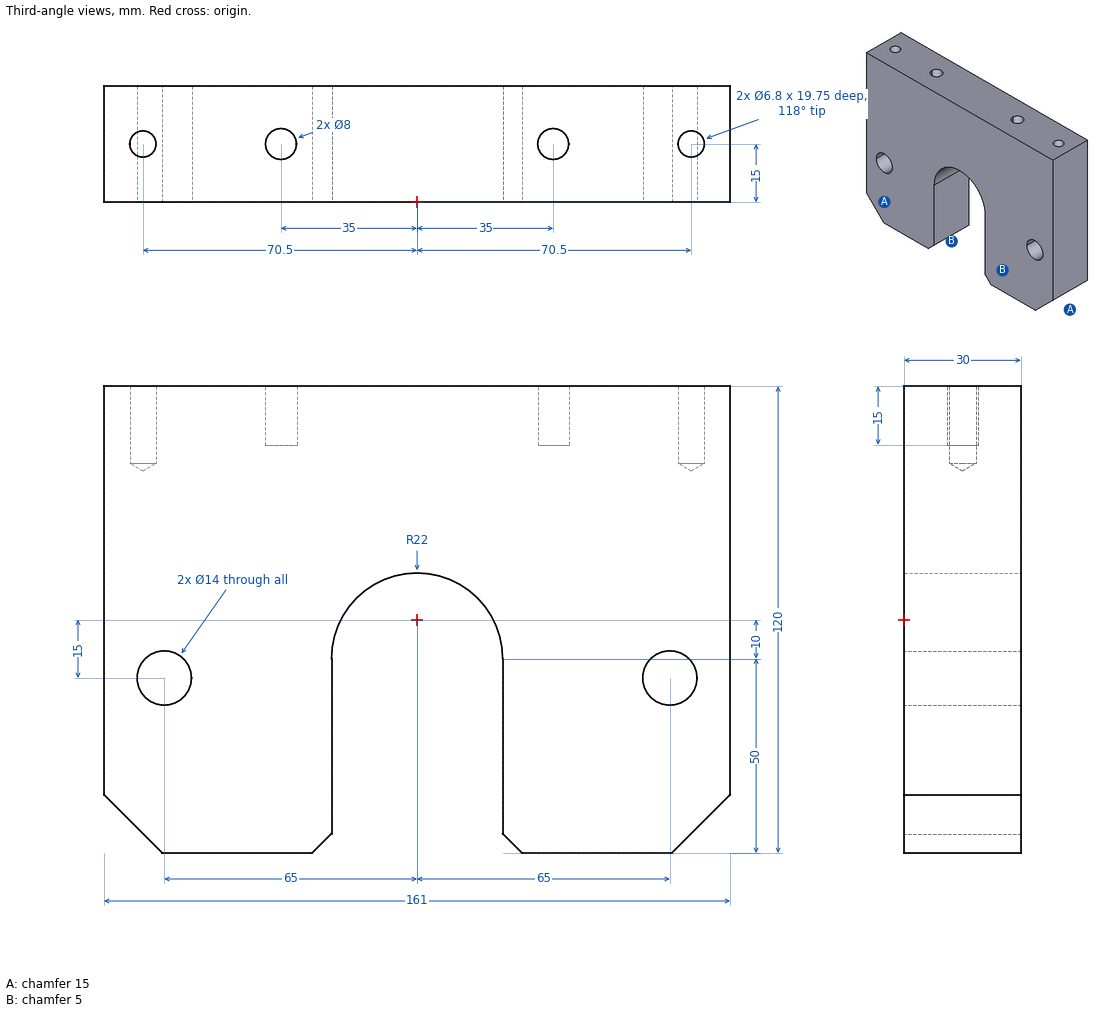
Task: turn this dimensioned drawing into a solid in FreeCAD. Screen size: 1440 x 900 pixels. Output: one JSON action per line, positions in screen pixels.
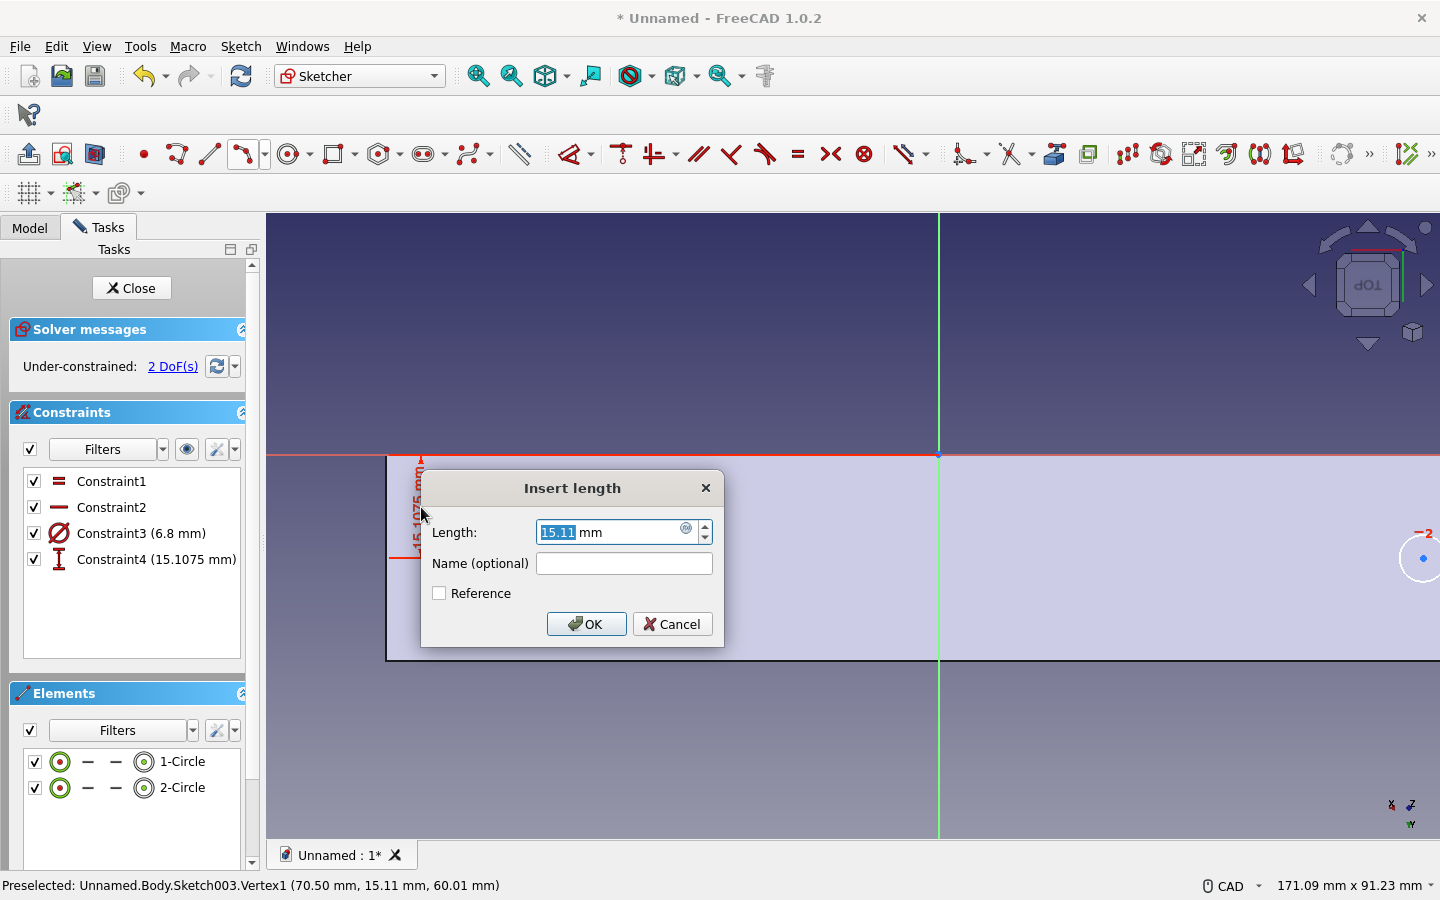
{"action": "type", "text": "15"}
{"action": "key", "text": "Return"}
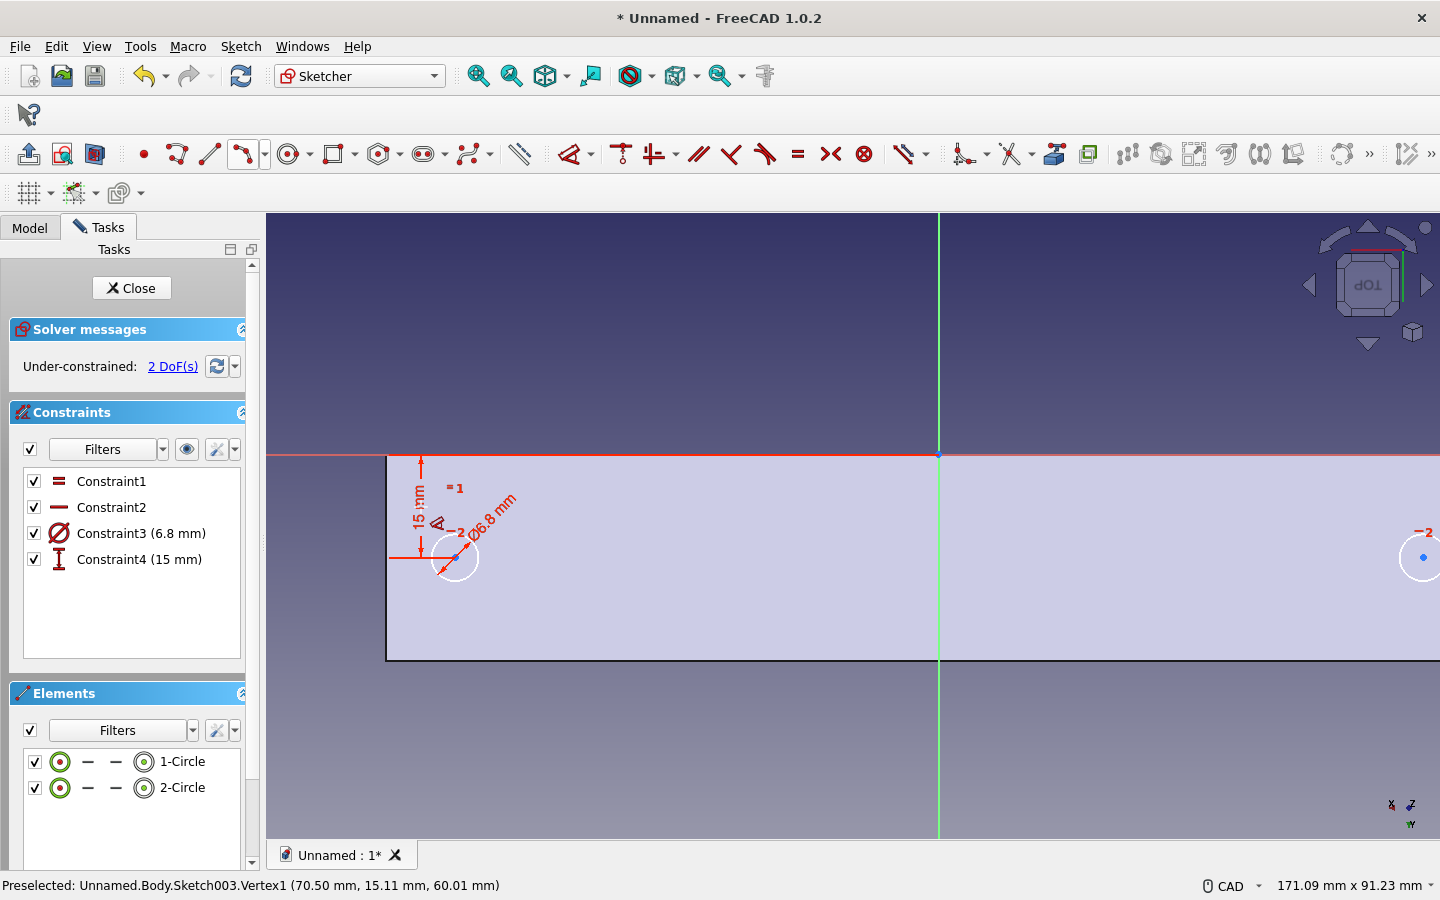
{"action": "left_click", "coordinate": [455, 558]}
{"action": "left_click", "coordinate": [697, 421]}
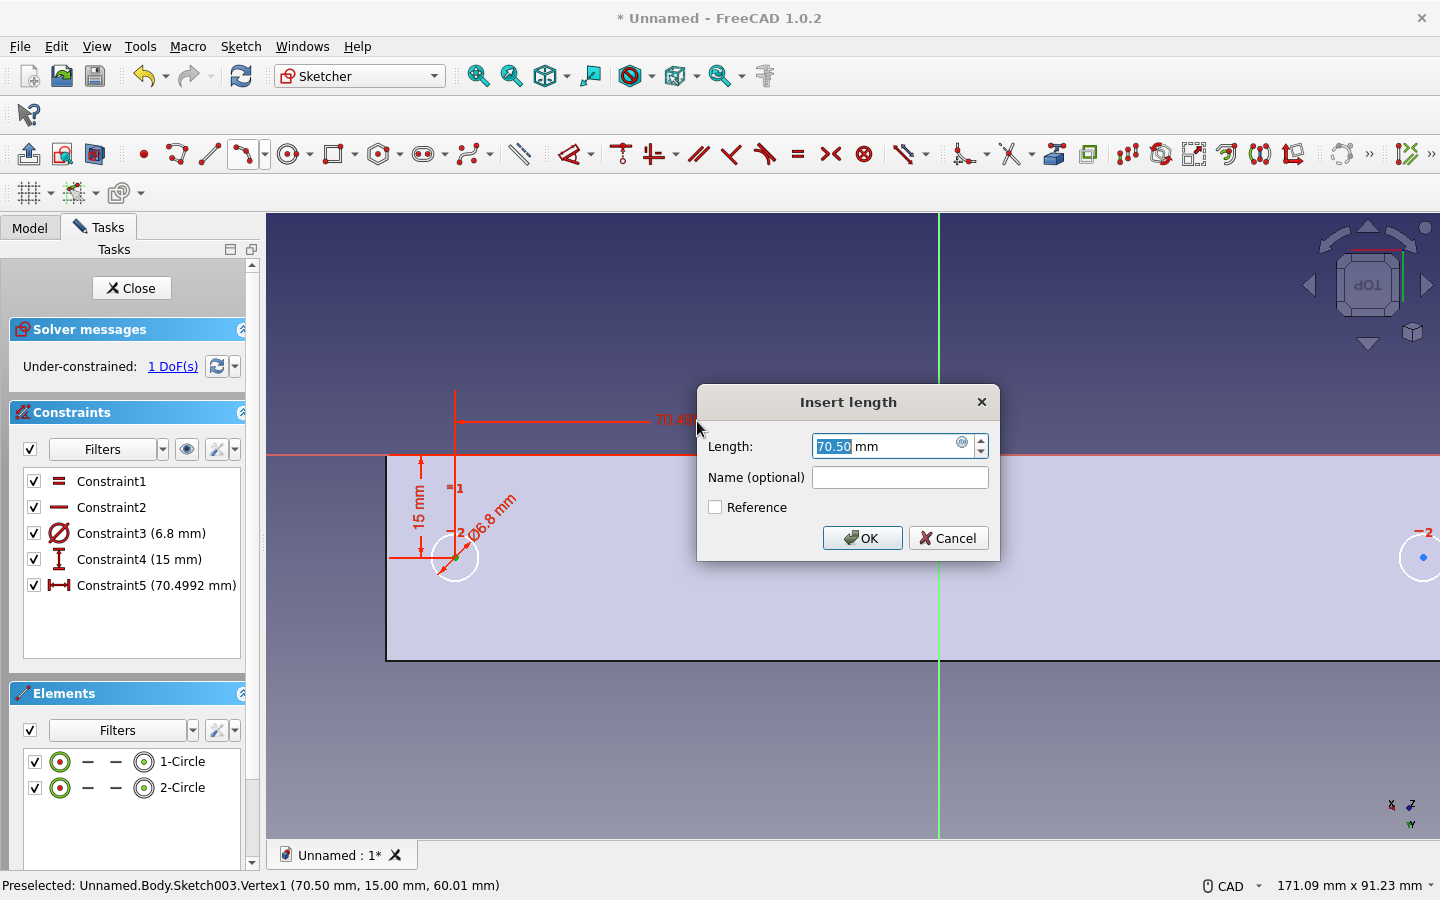
{"action": "type", "text": "70.5"}
{"action": "key", "text": "Return"}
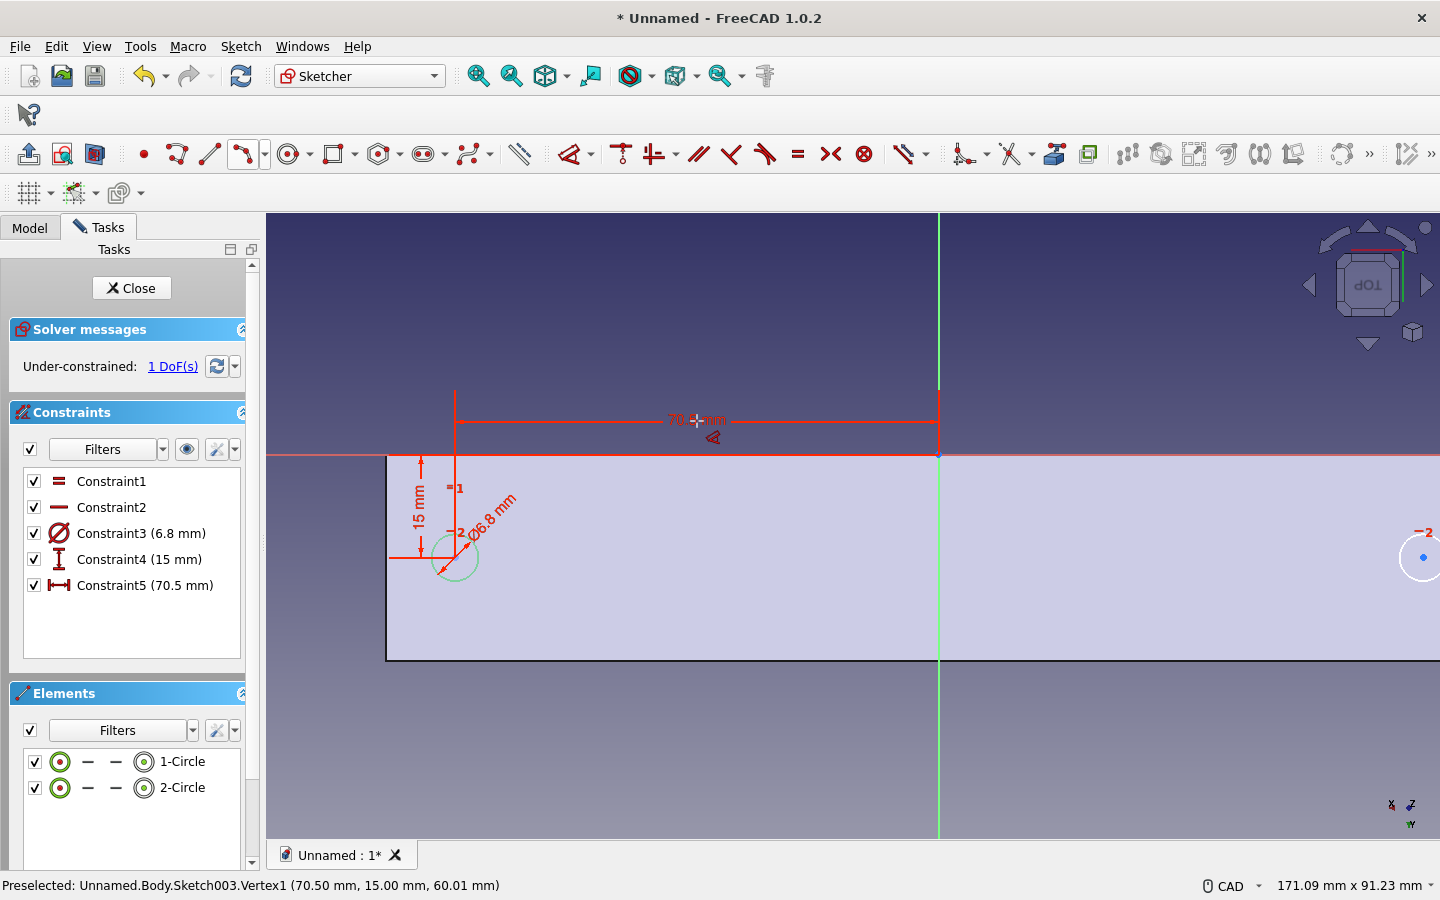
{"action": "scroll", "coordinate": [471, 543], "scroll_direction": "down", "scroll_amount": 2}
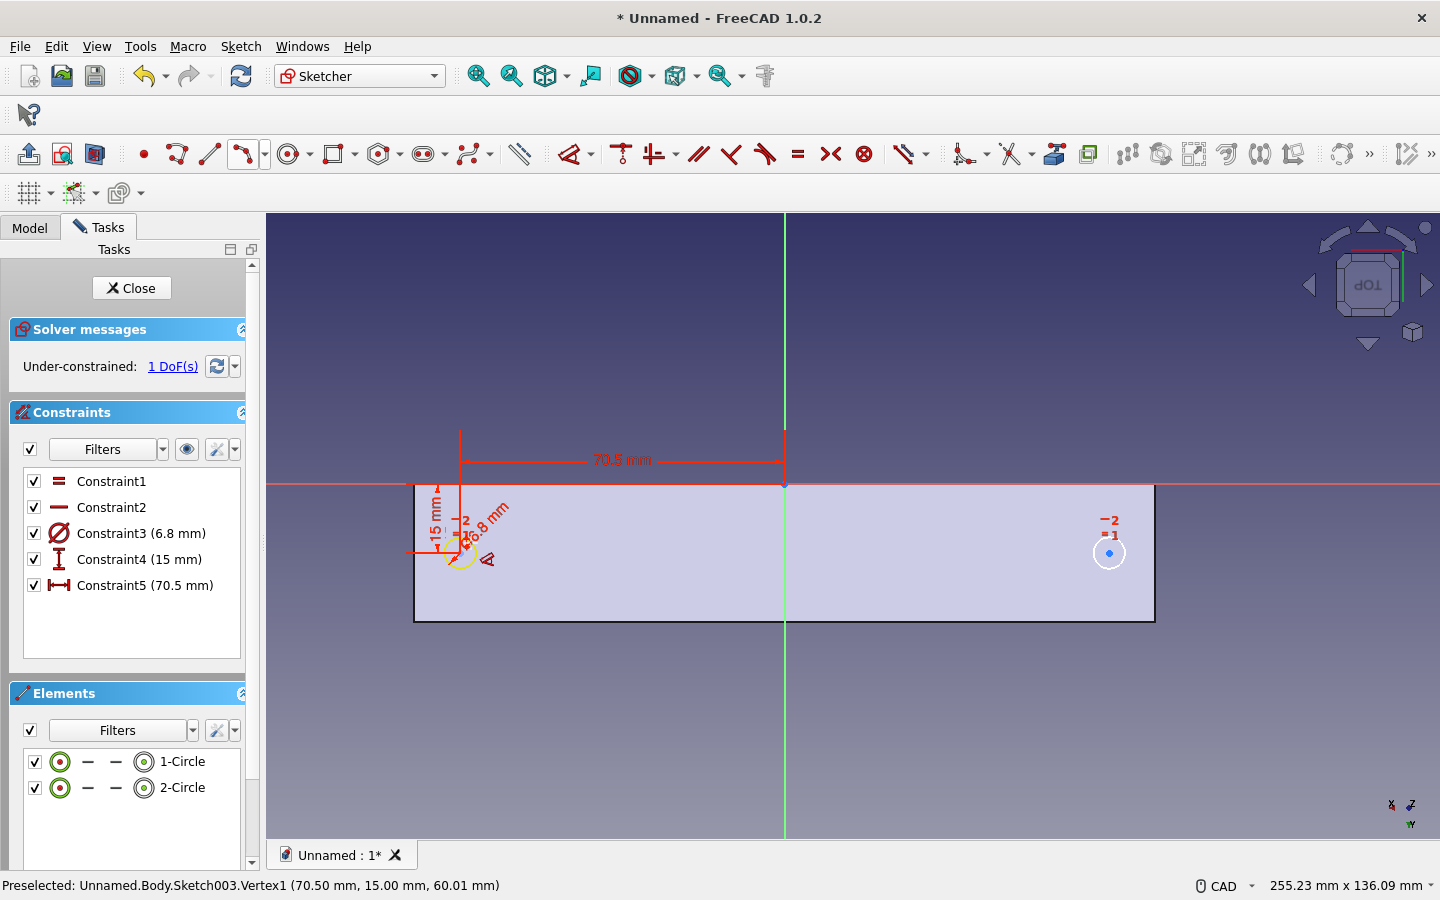
{"action": "left_click", "coordinate": [1109, 553]}
{"action": "left_click", "coordinate": [947, 450]}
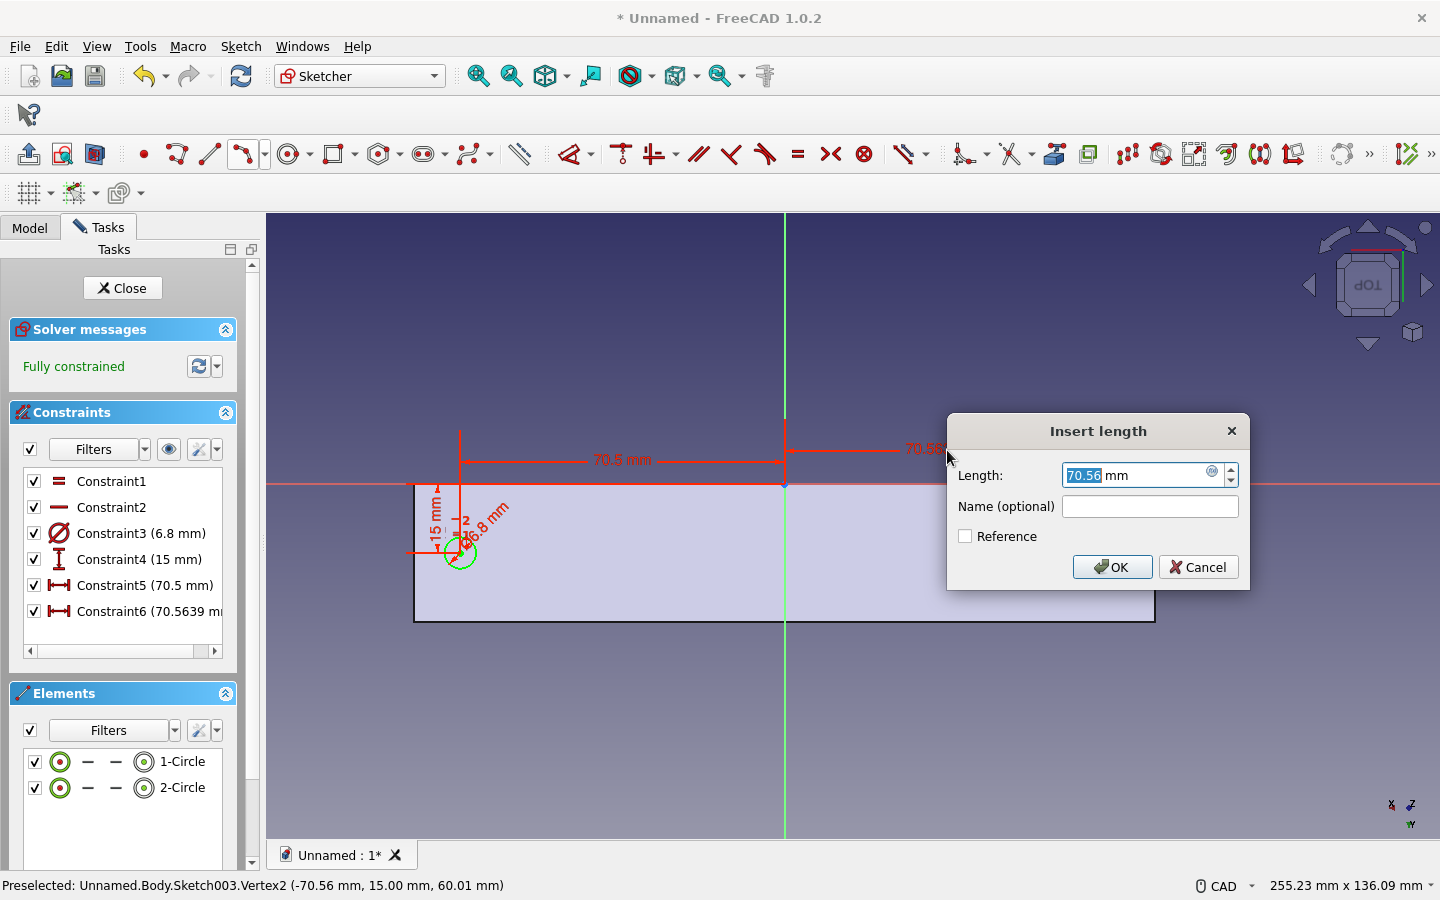
{"action": "type", "text": "70.5"}
{"action": "key", "text": "Return"}
{"action": "key", "text": "Escape"}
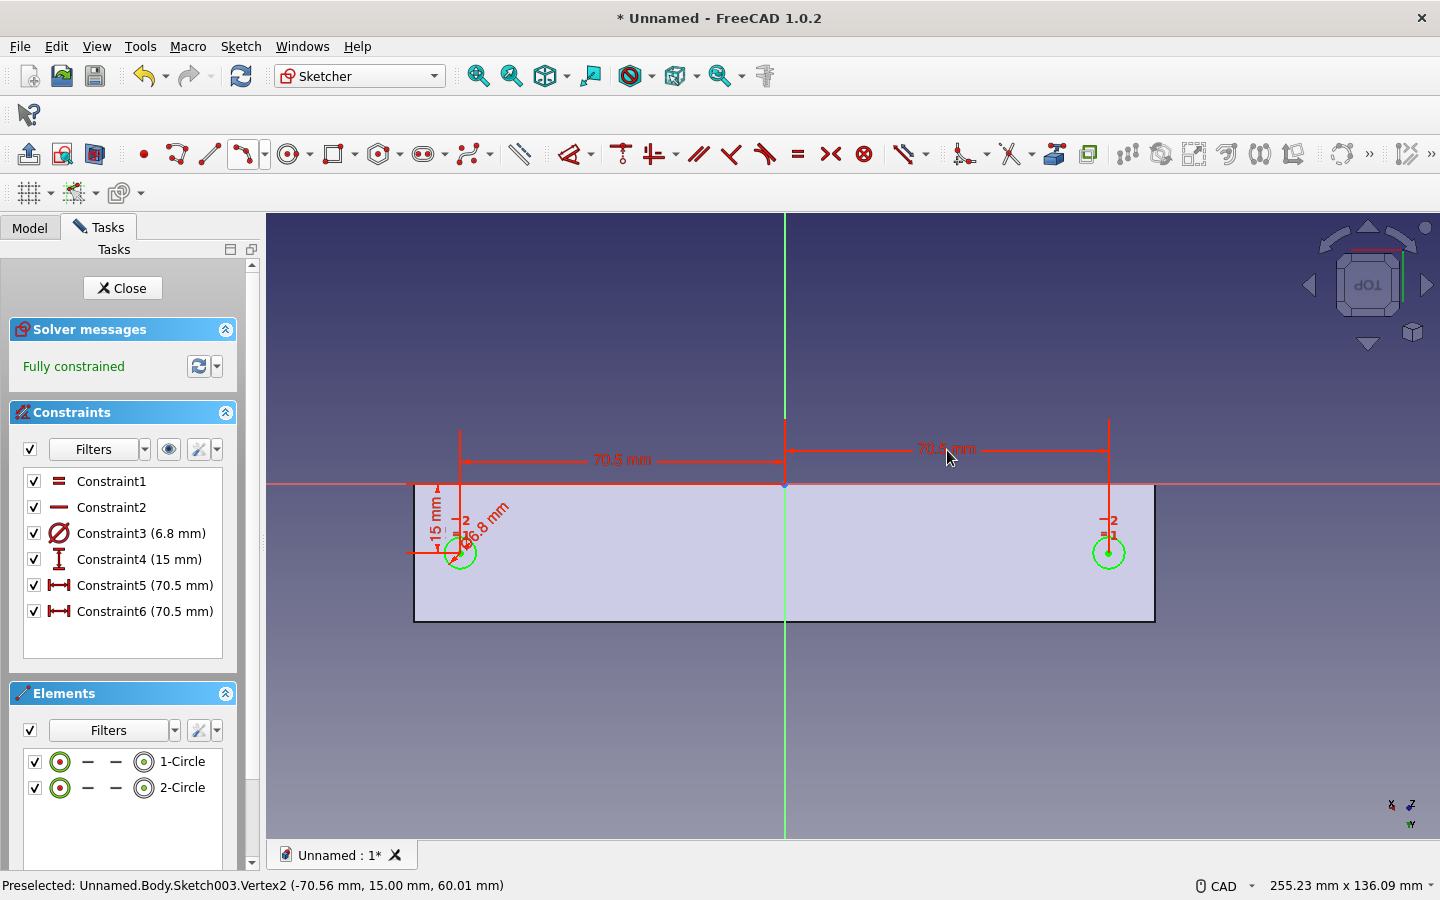
{"action": "left_click", "coordinate": [123, 288]}